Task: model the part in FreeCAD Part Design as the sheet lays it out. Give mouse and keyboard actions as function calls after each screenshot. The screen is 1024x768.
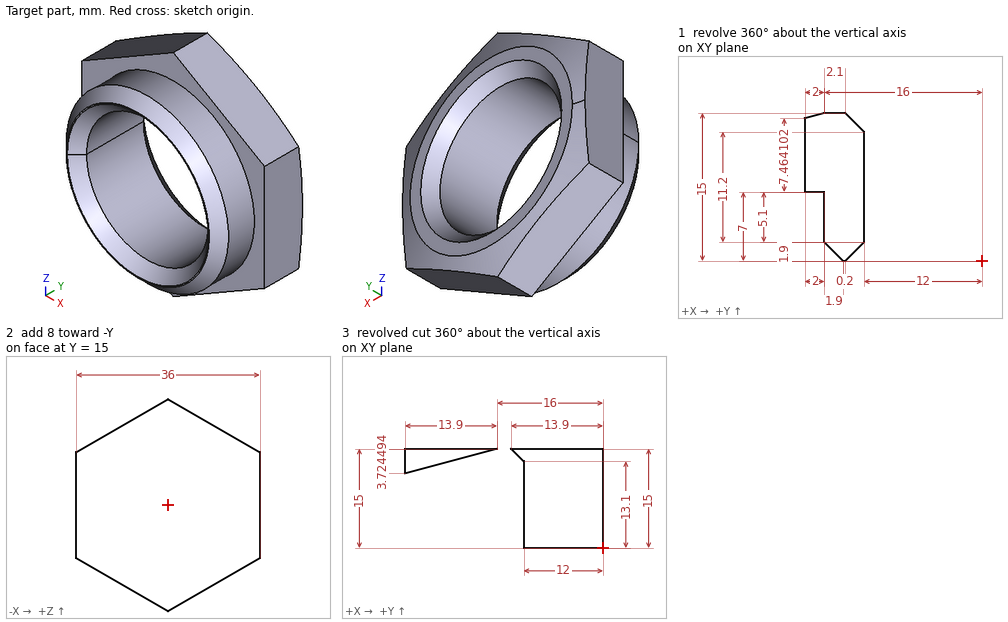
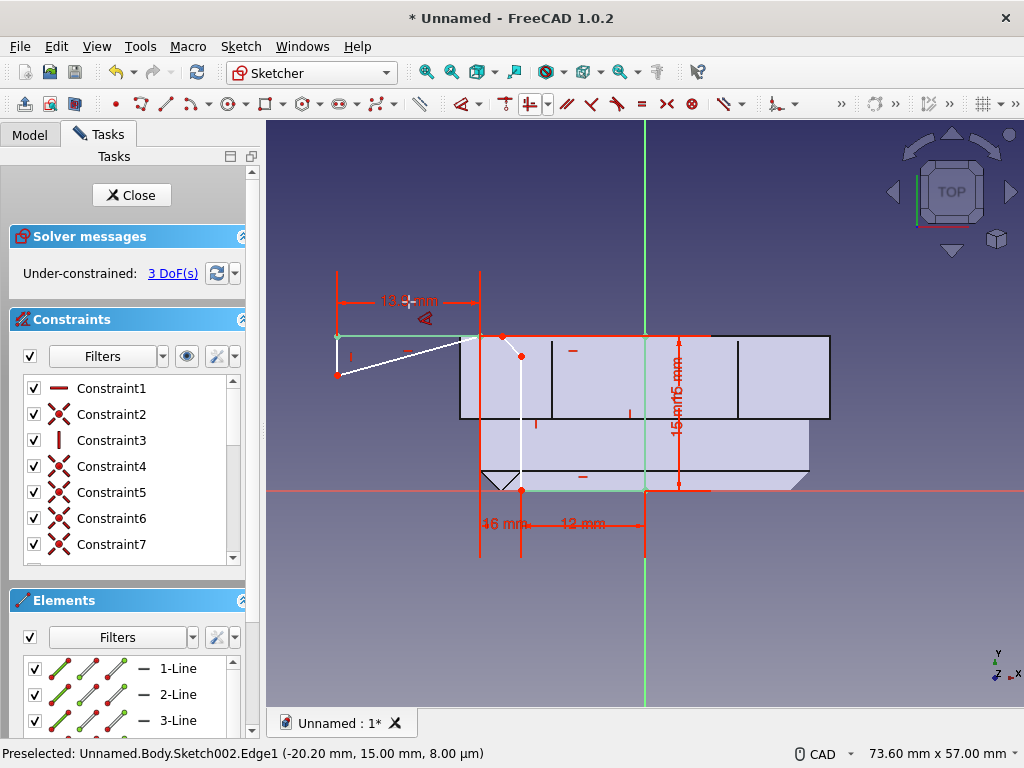
click(602, 336)
click(574, 302)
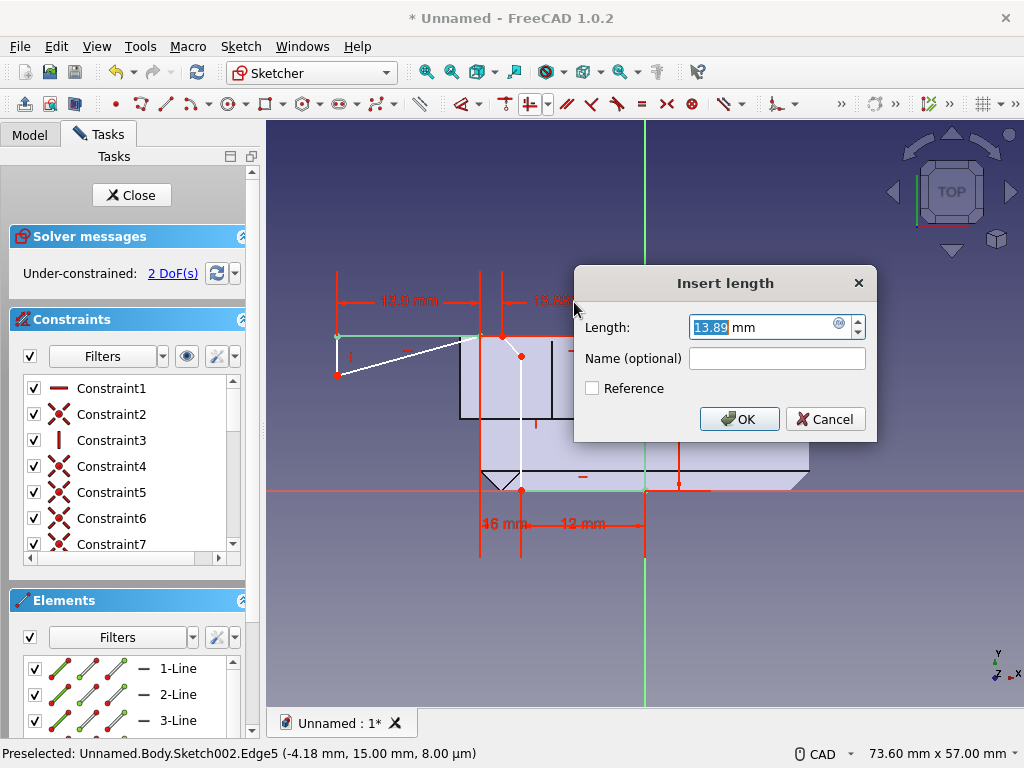
text(13.9)
key(Return)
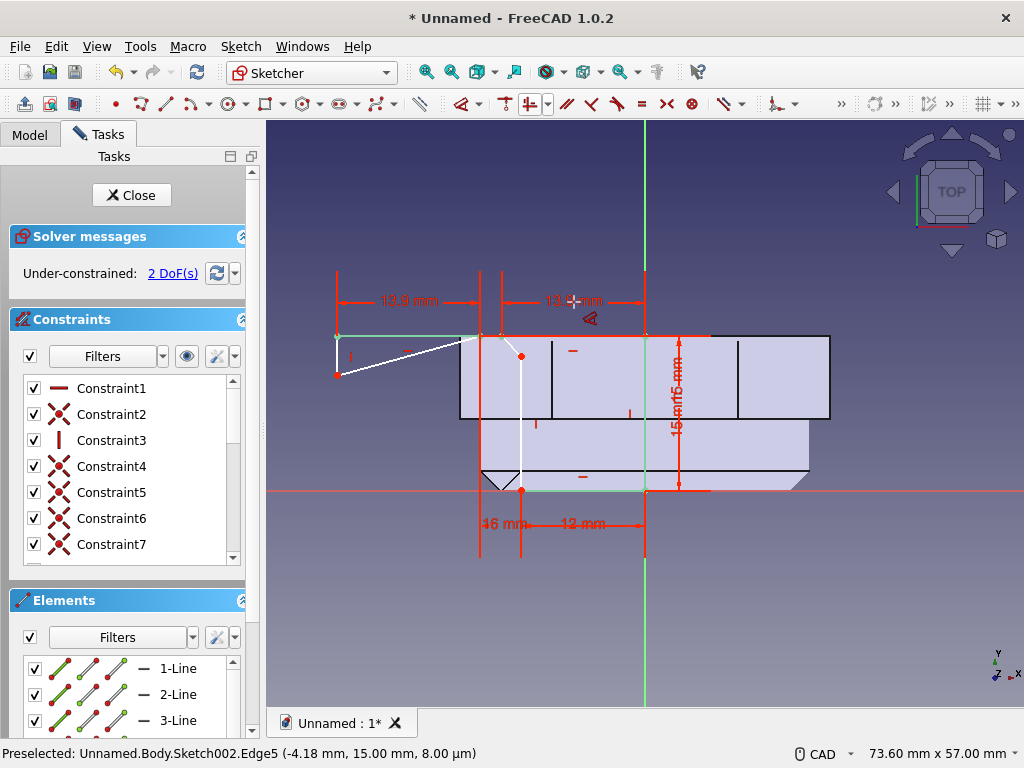
click(521, 397)
click(555, 424)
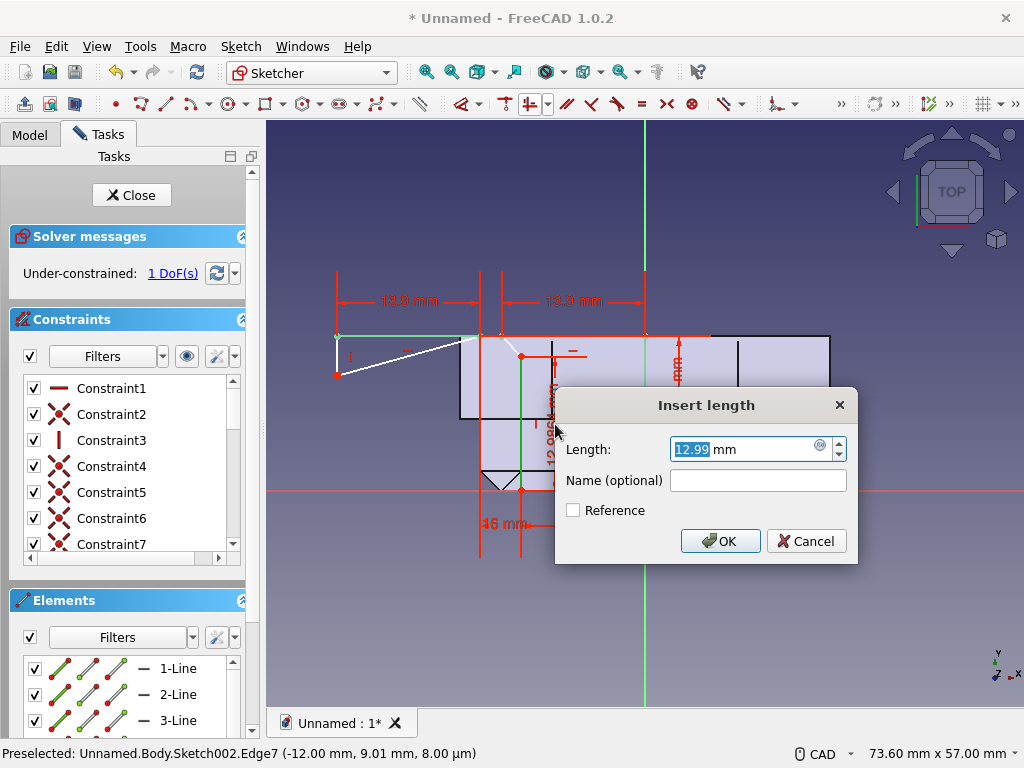
text(13.1)
key(Return)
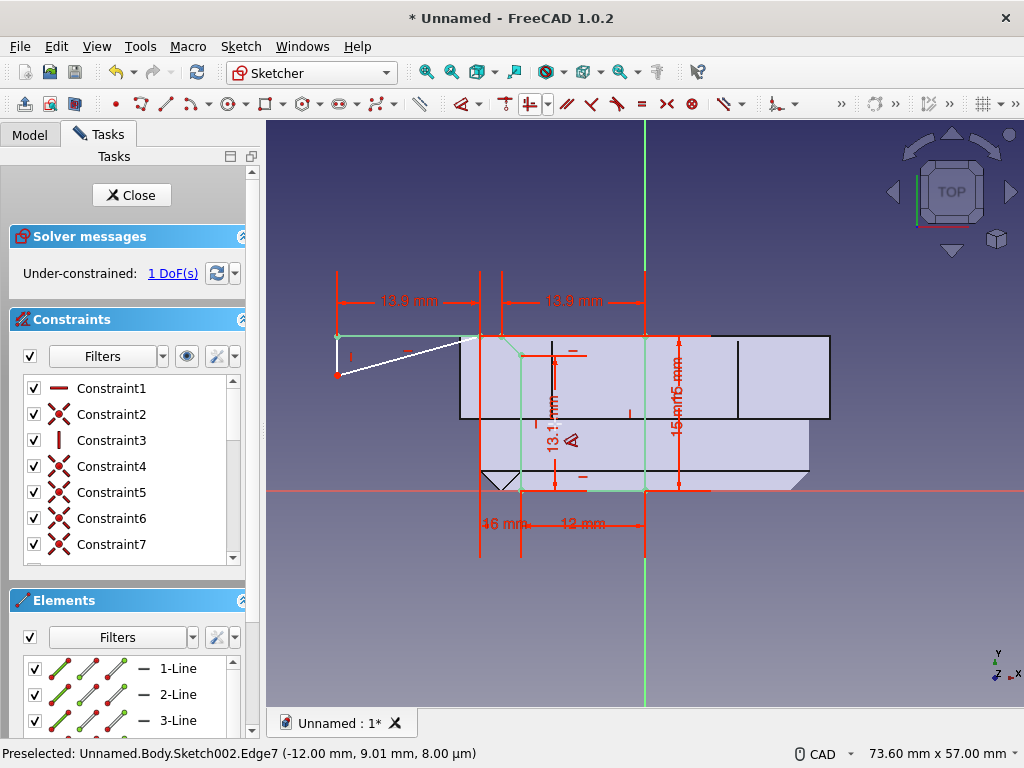
click(337, 348)
click(303, 356)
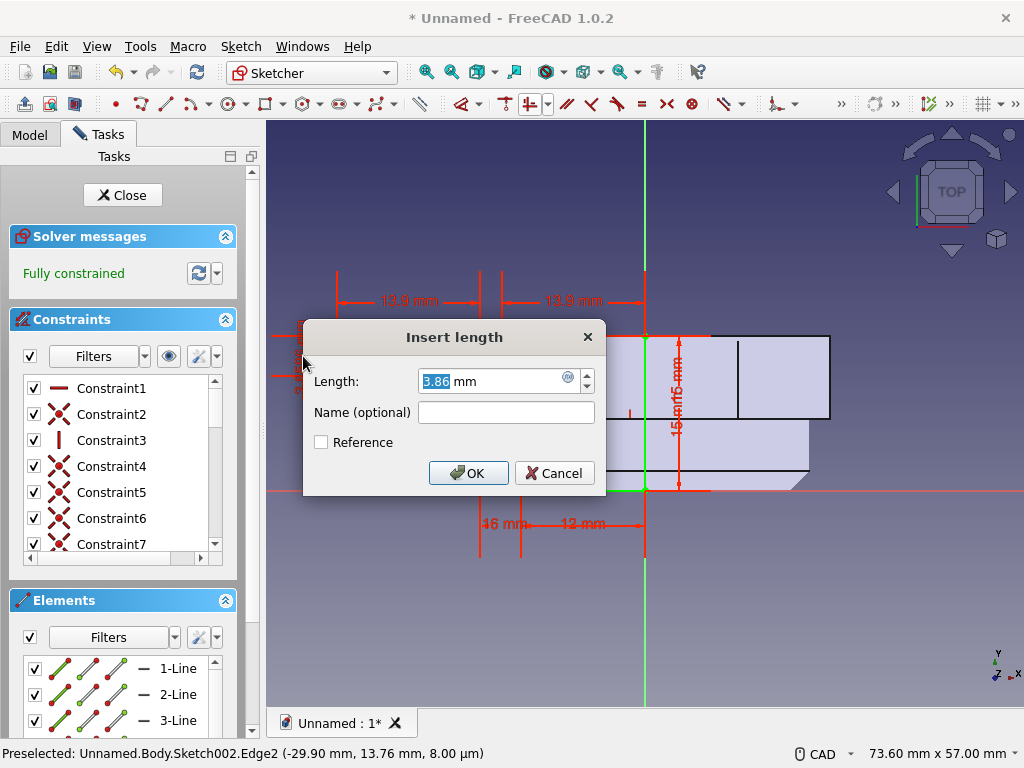
text(3.724494)
key(Return)
key(Escape)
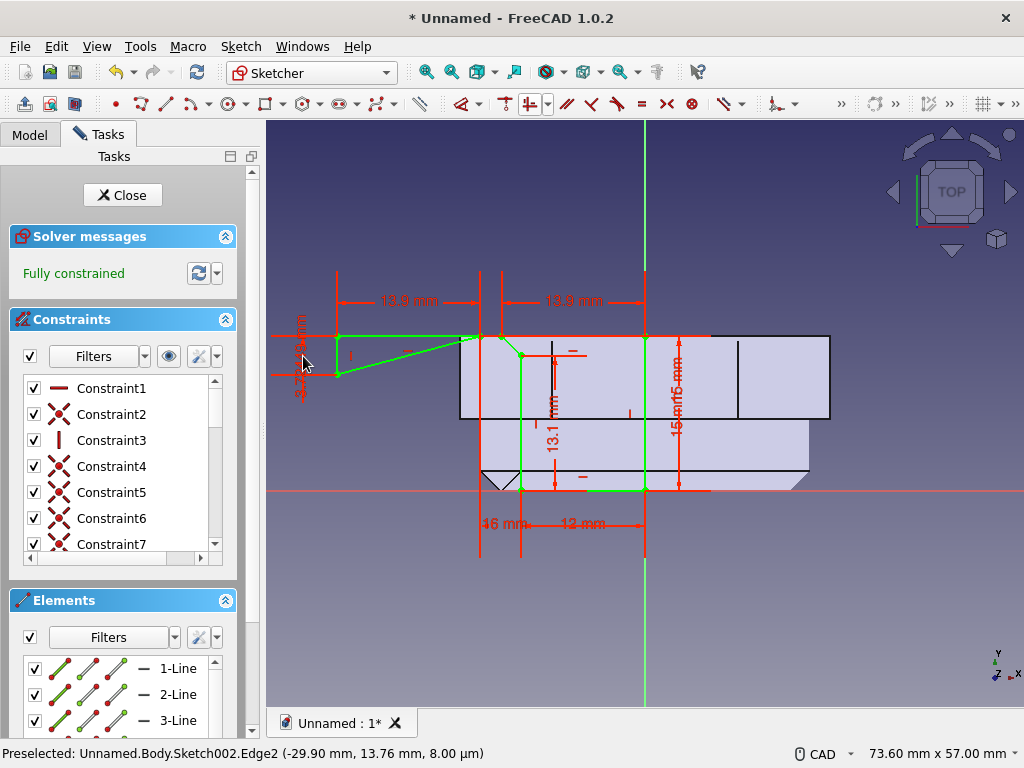
click(123, 195)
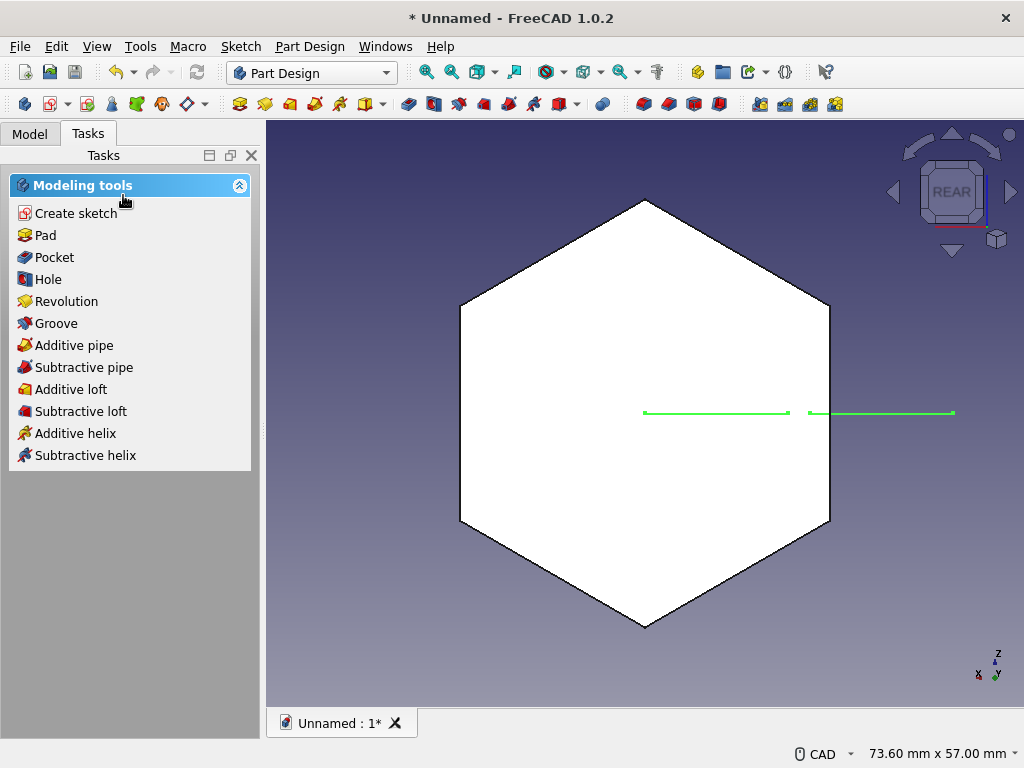
click(459, 104)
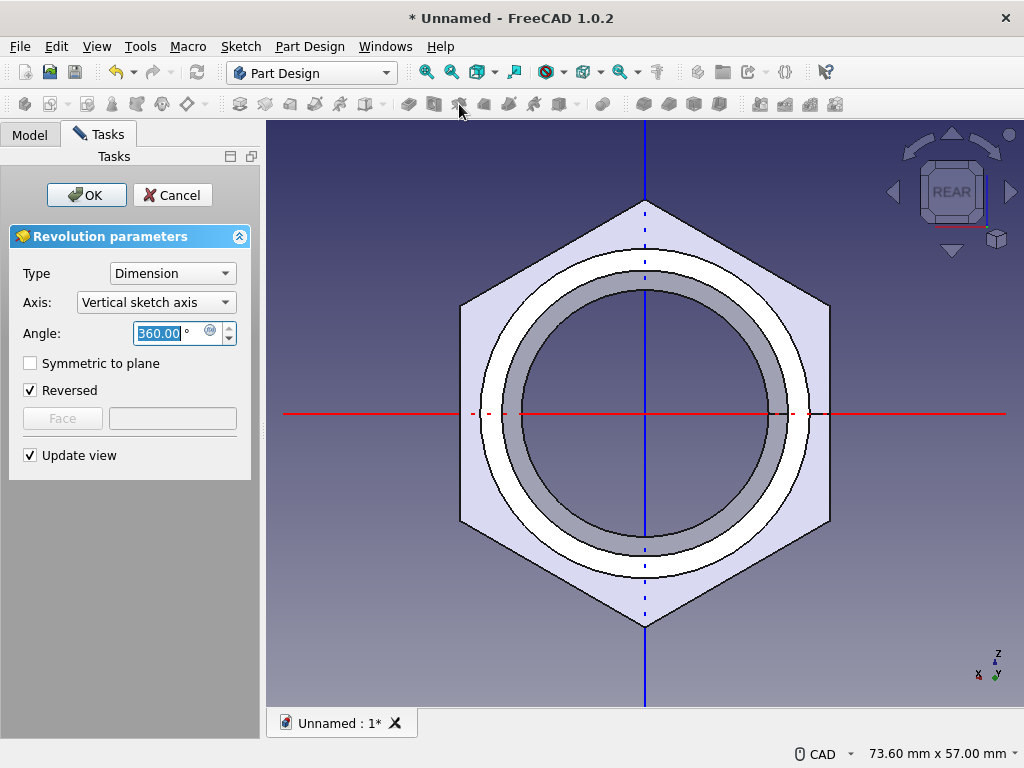
click(87, 195)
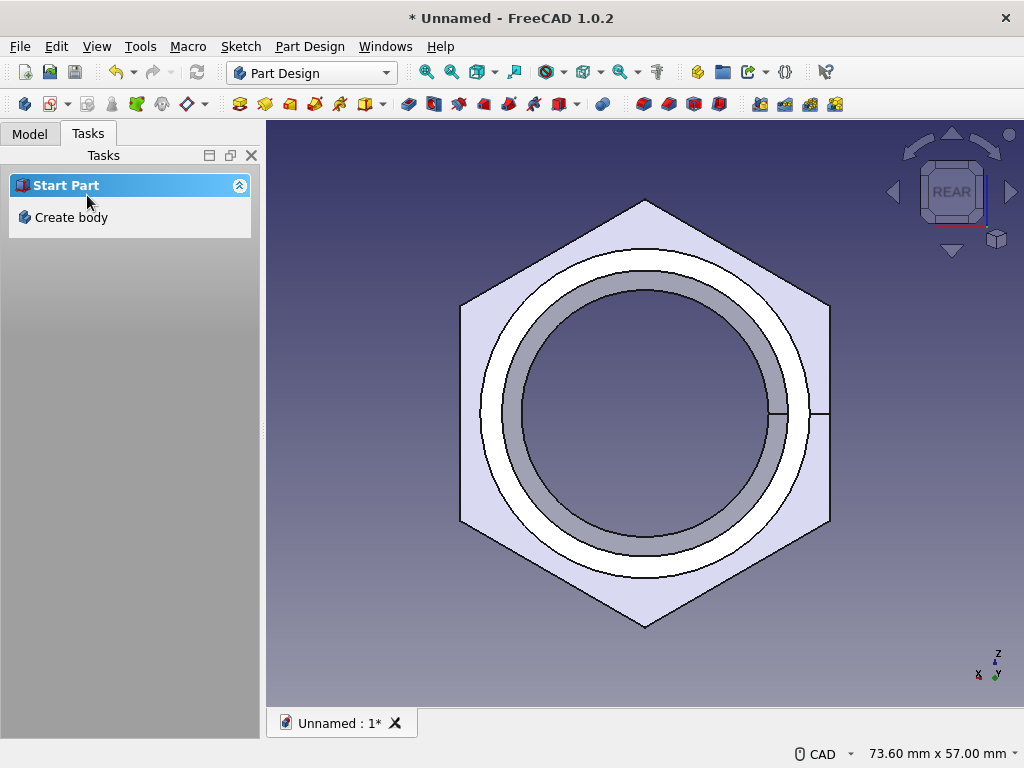
key(0)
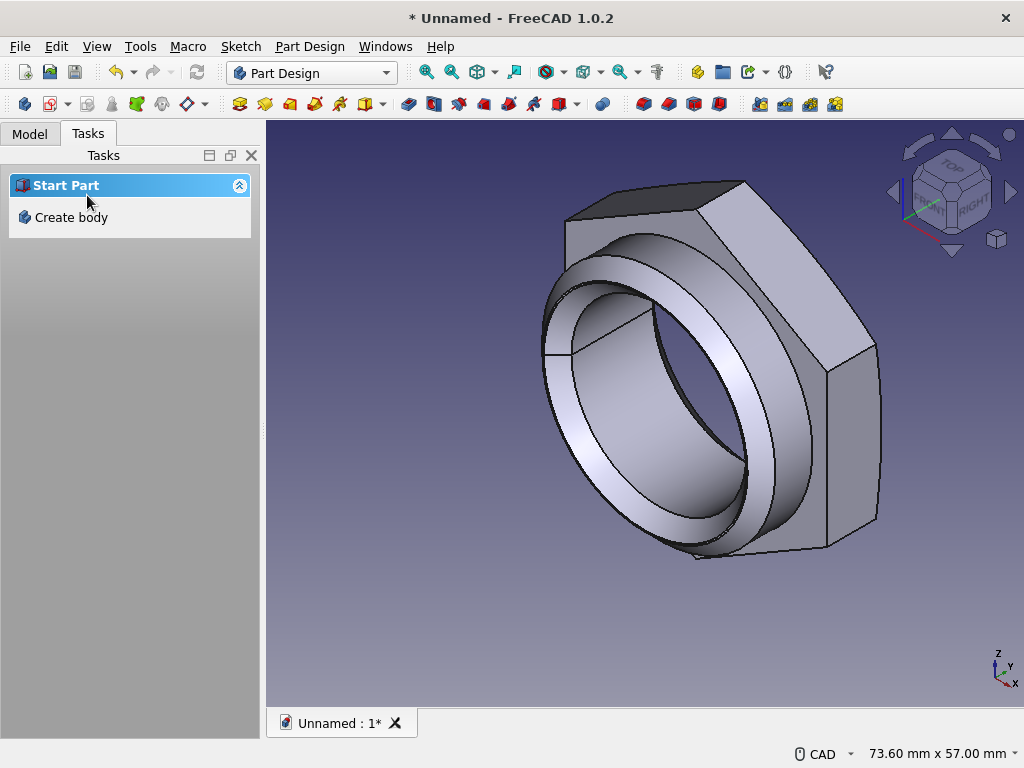
key(v)
key(f)